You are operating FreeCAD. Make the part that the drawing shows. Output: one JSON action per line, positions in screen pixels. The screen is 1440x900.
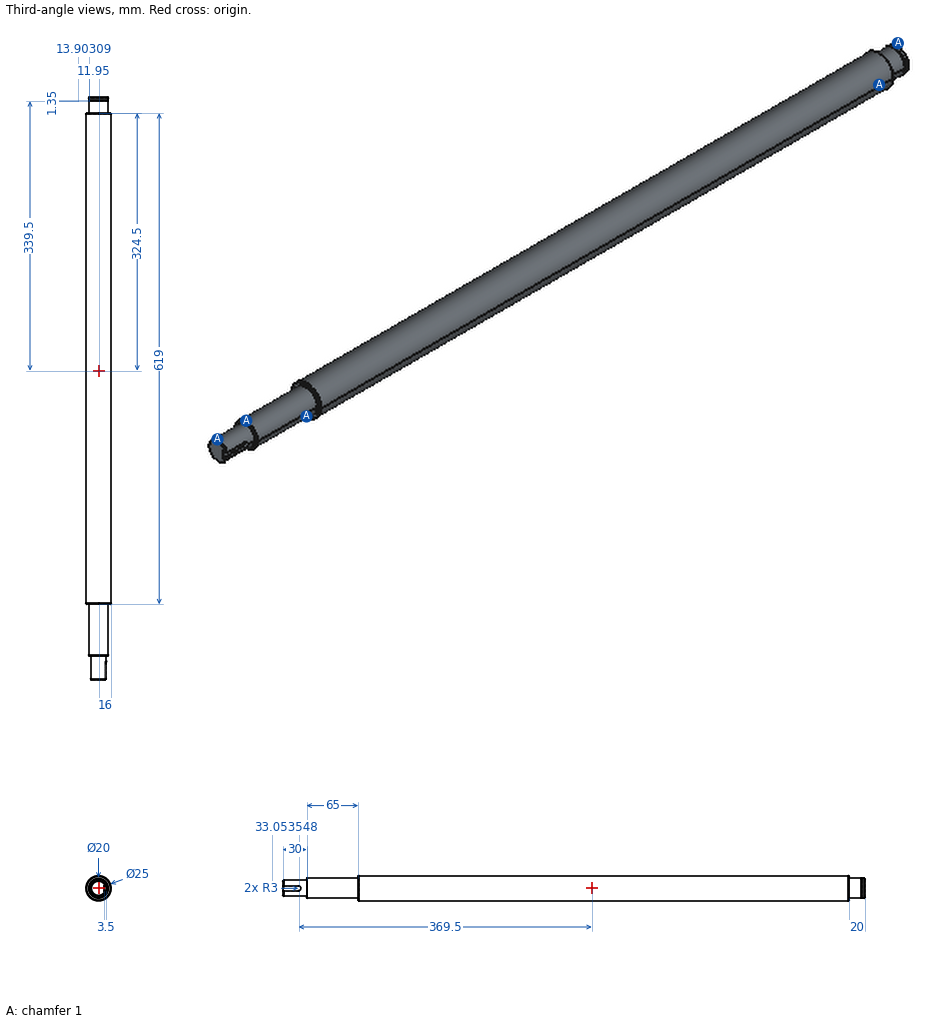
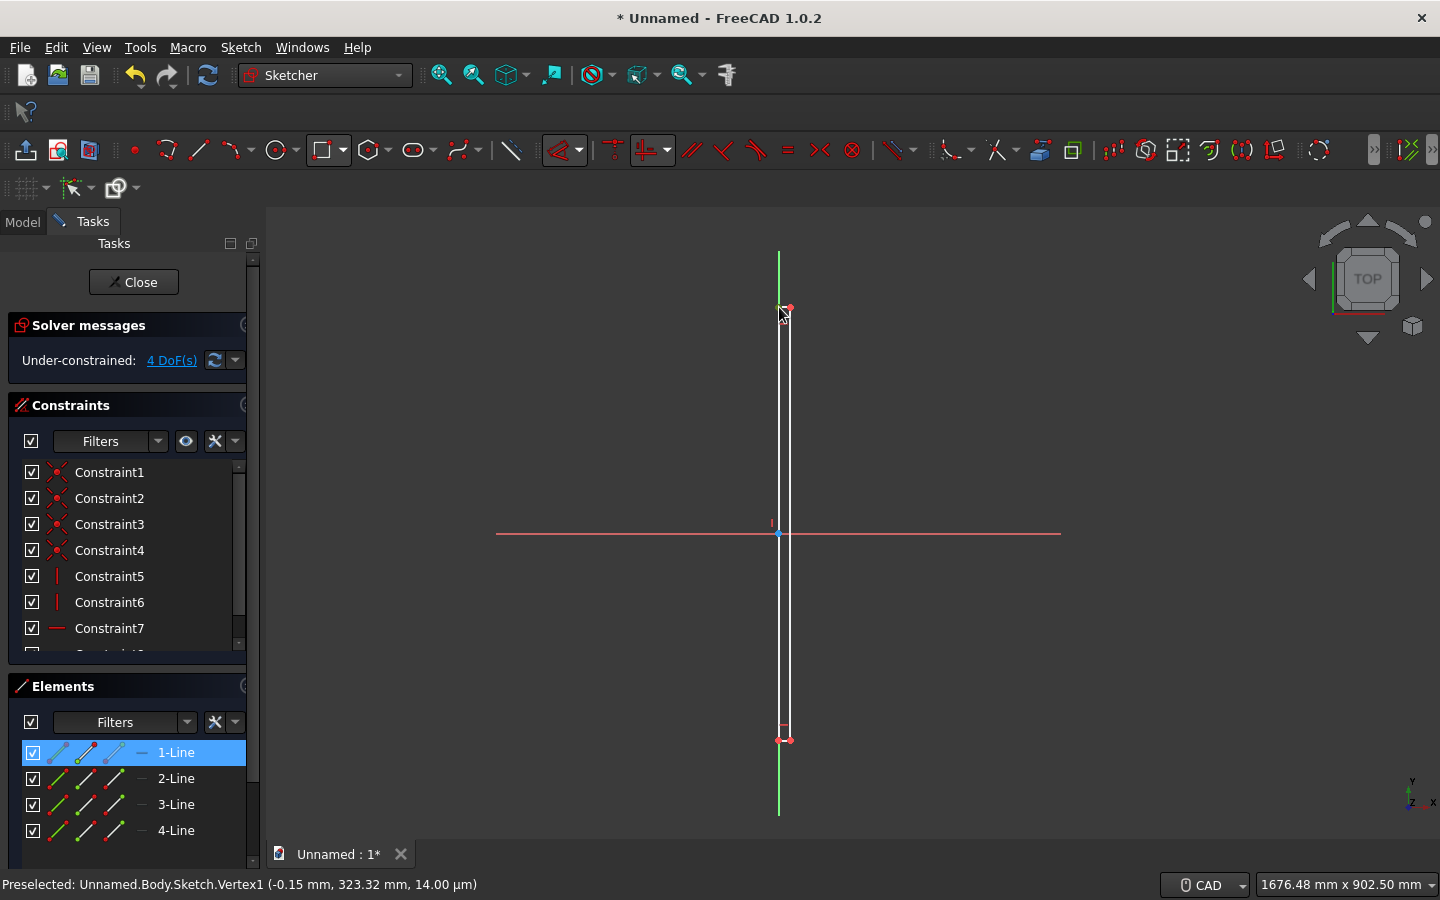
{"action": "left_click", "coordinate": [779, 276]}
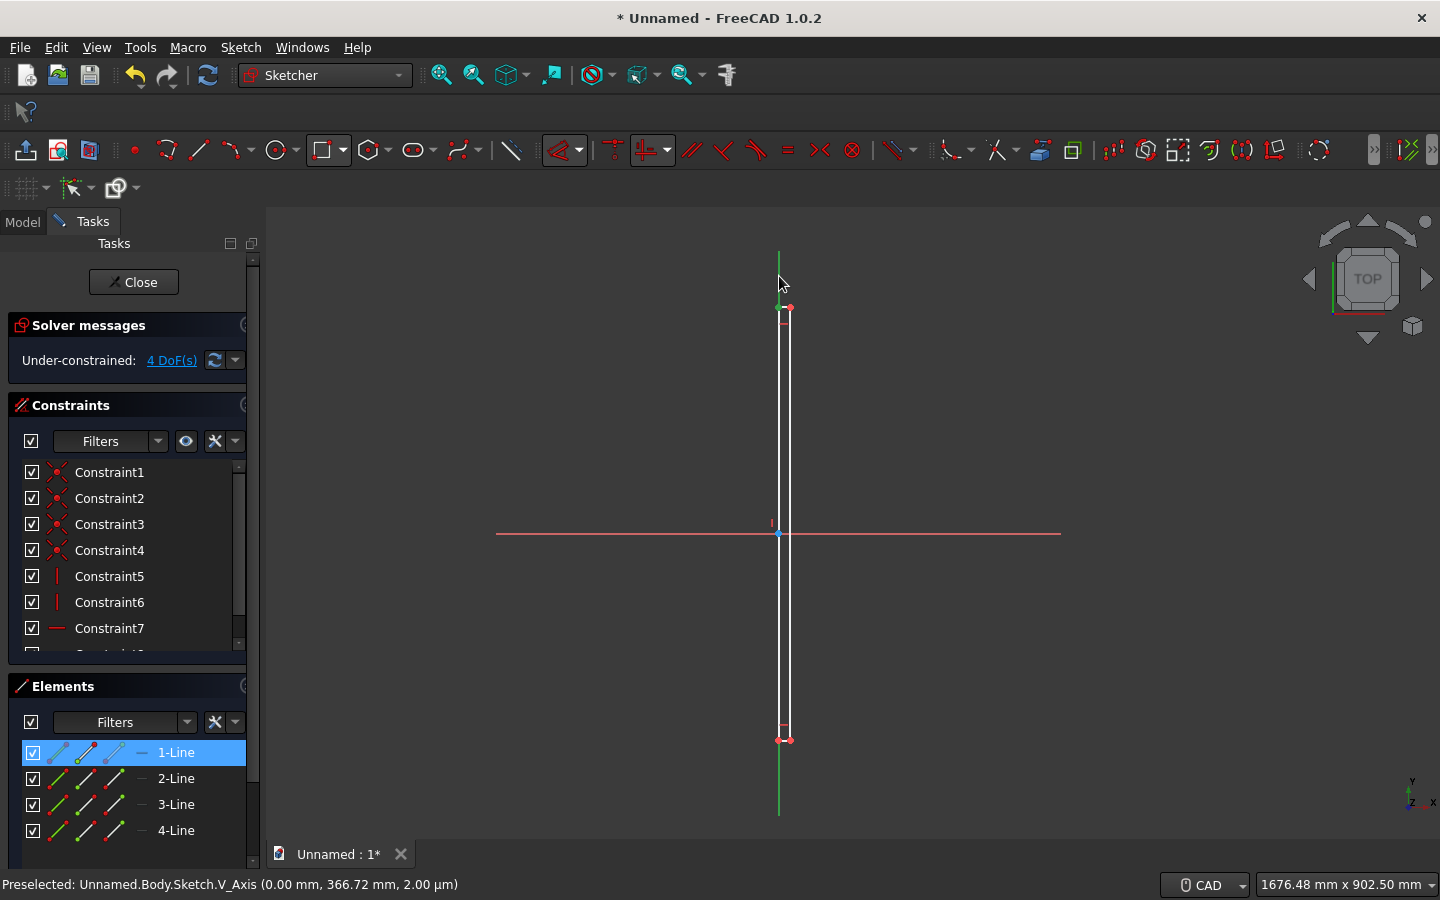
{"action": "left_click", "coordinate": [614, 150]}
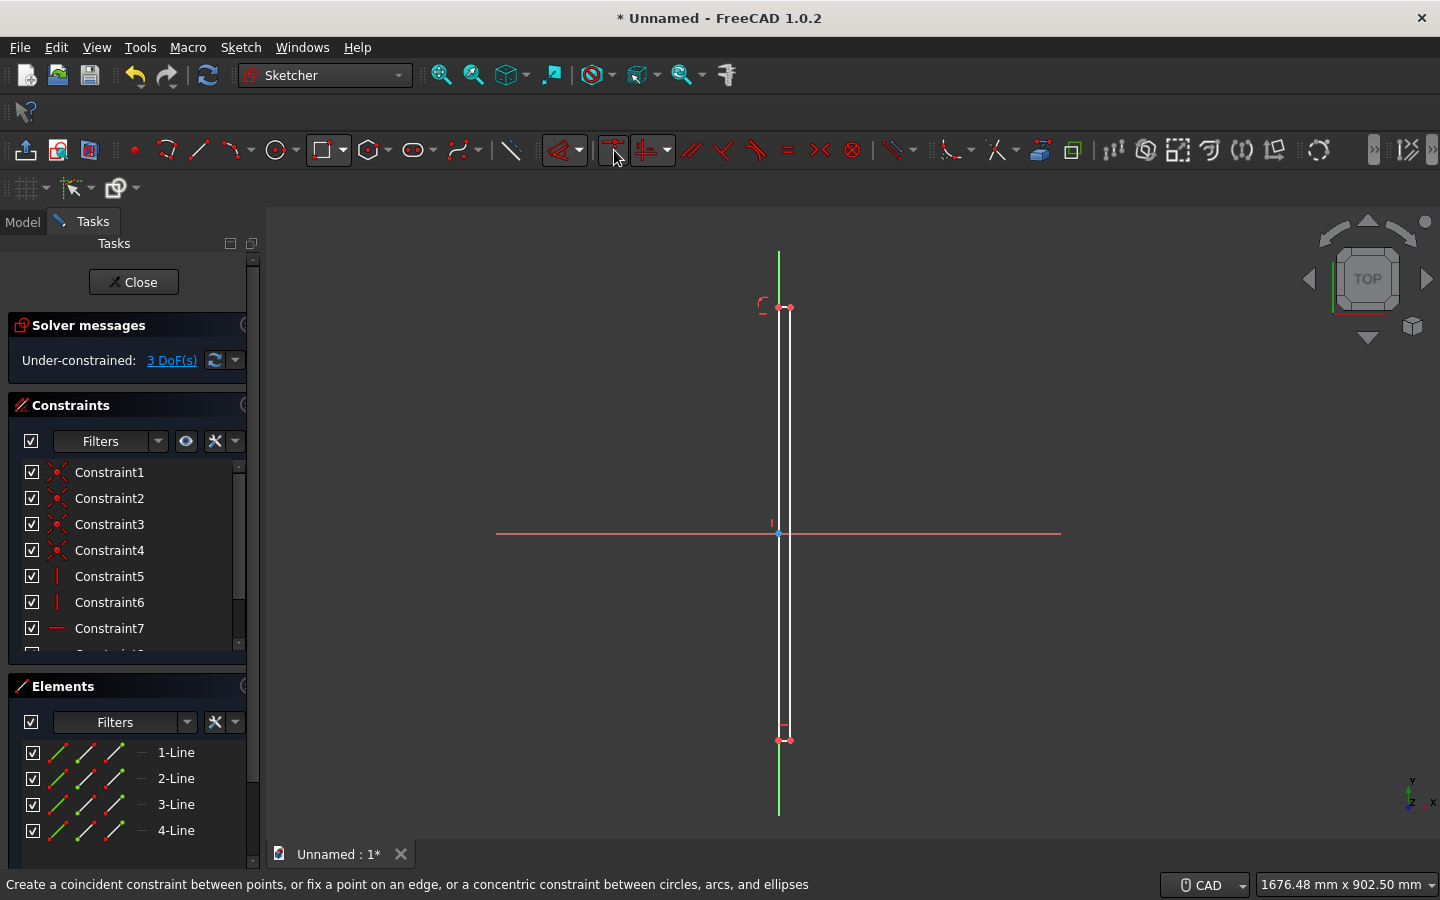
{"action": "left_click", "coordinate": [558, 150]}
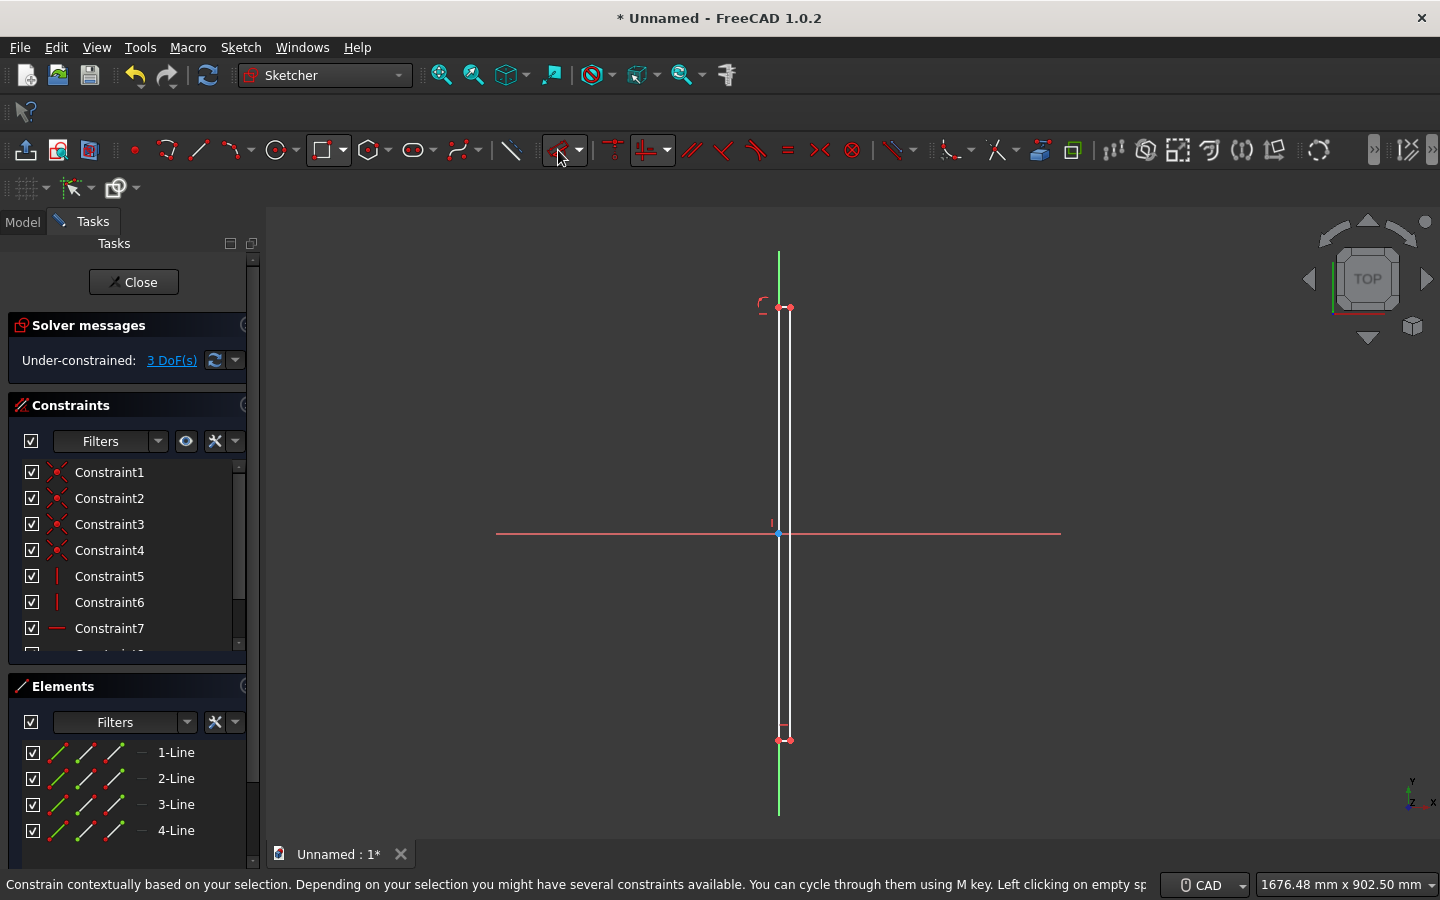
{"action": "scroll", "coordinate": [785, 741], "scroll_direction": "up", "scroll_amount": 7}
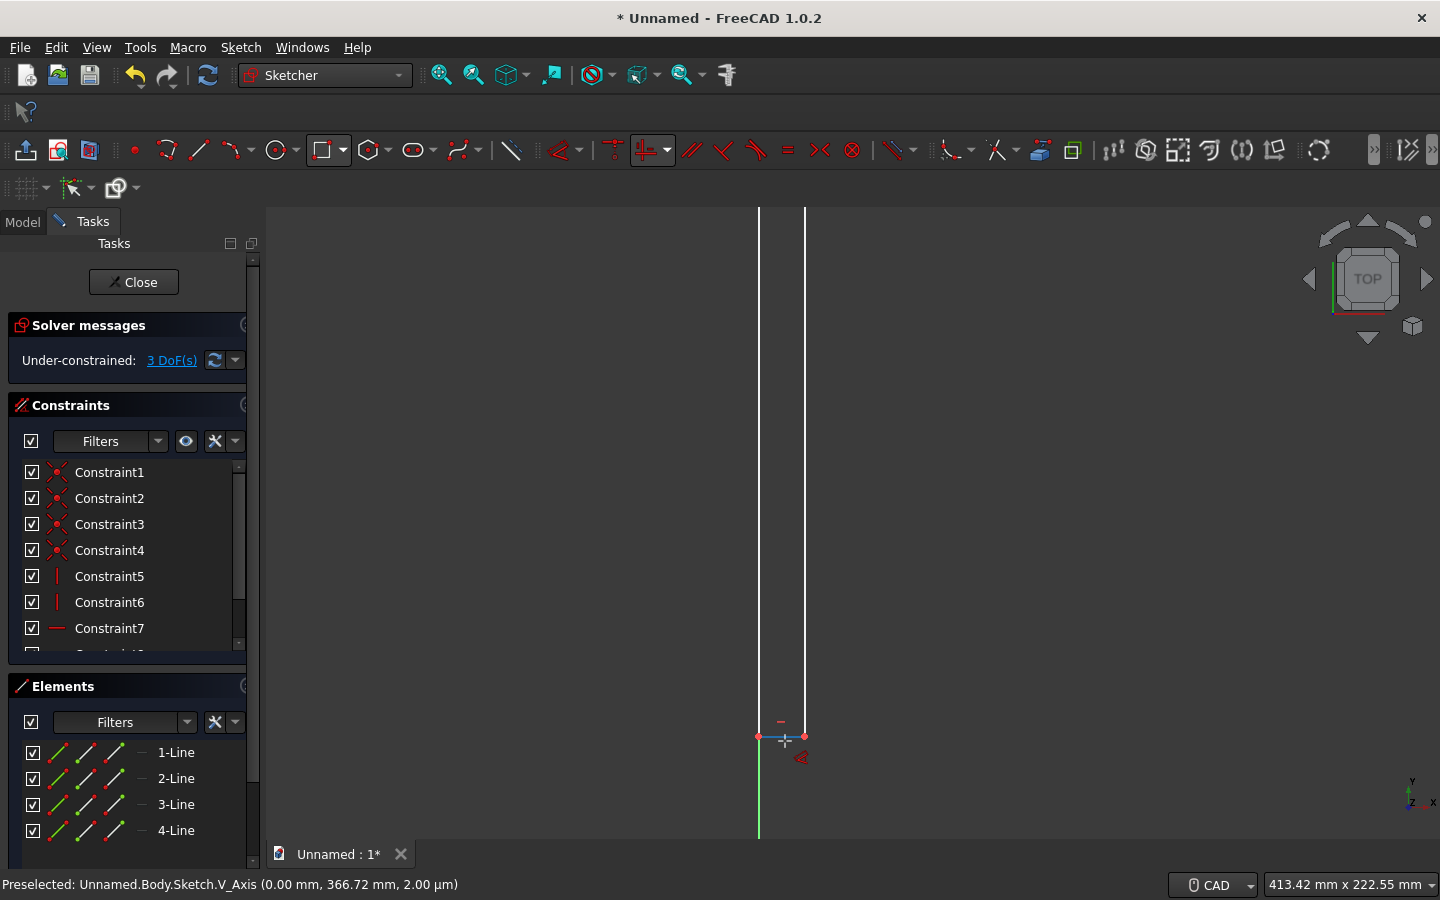
{"action": "left_click", "coordinate": [782, 737]}
{"action": "left_click", "coordinate": [782, 771]}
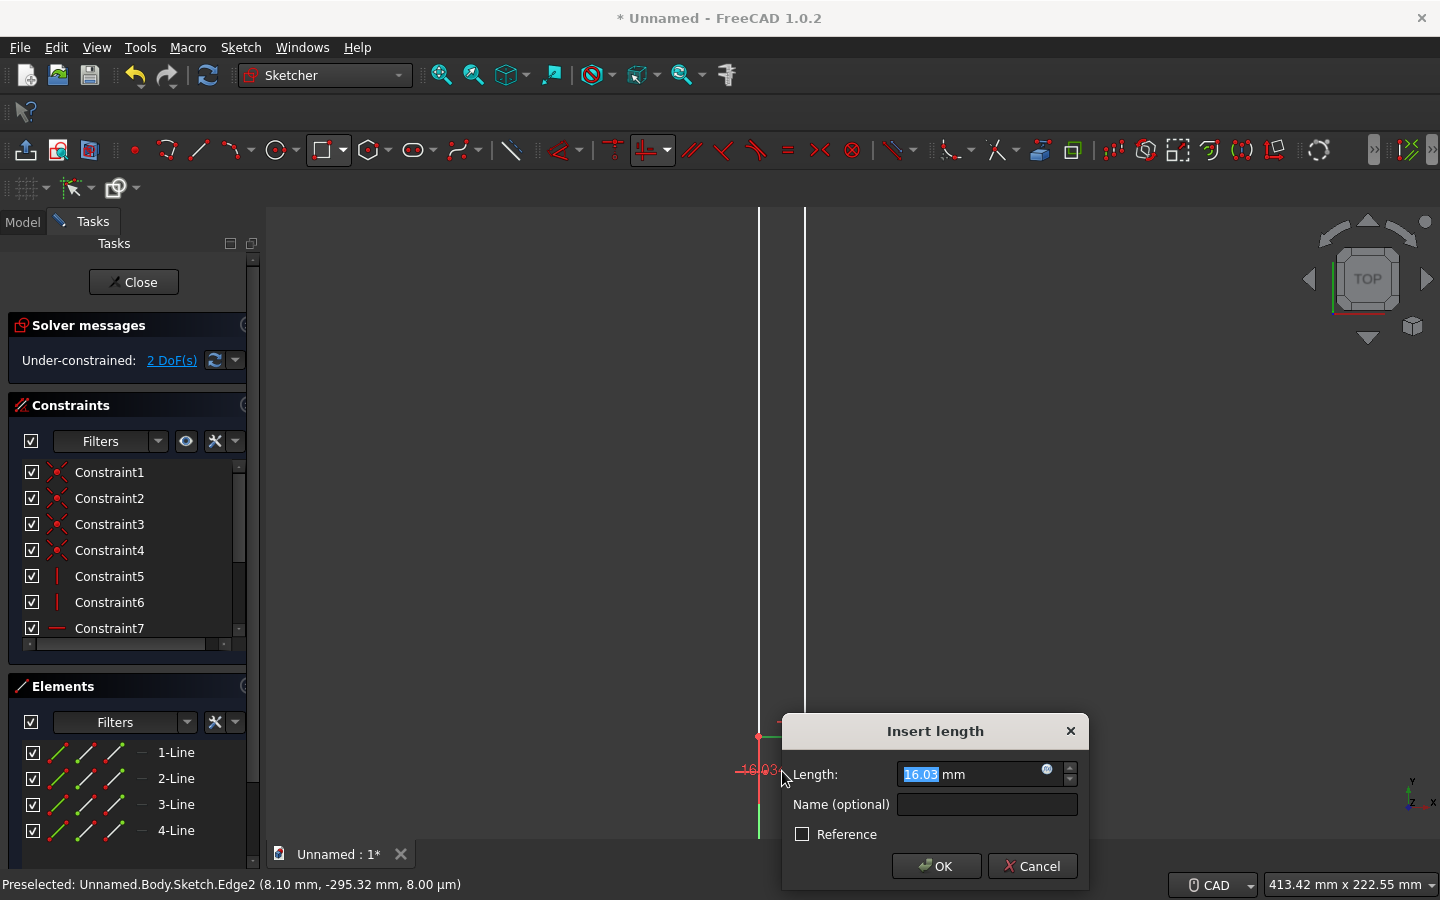
{"action": "type", "text": "16"}
{"action": "key", "text": "Return"}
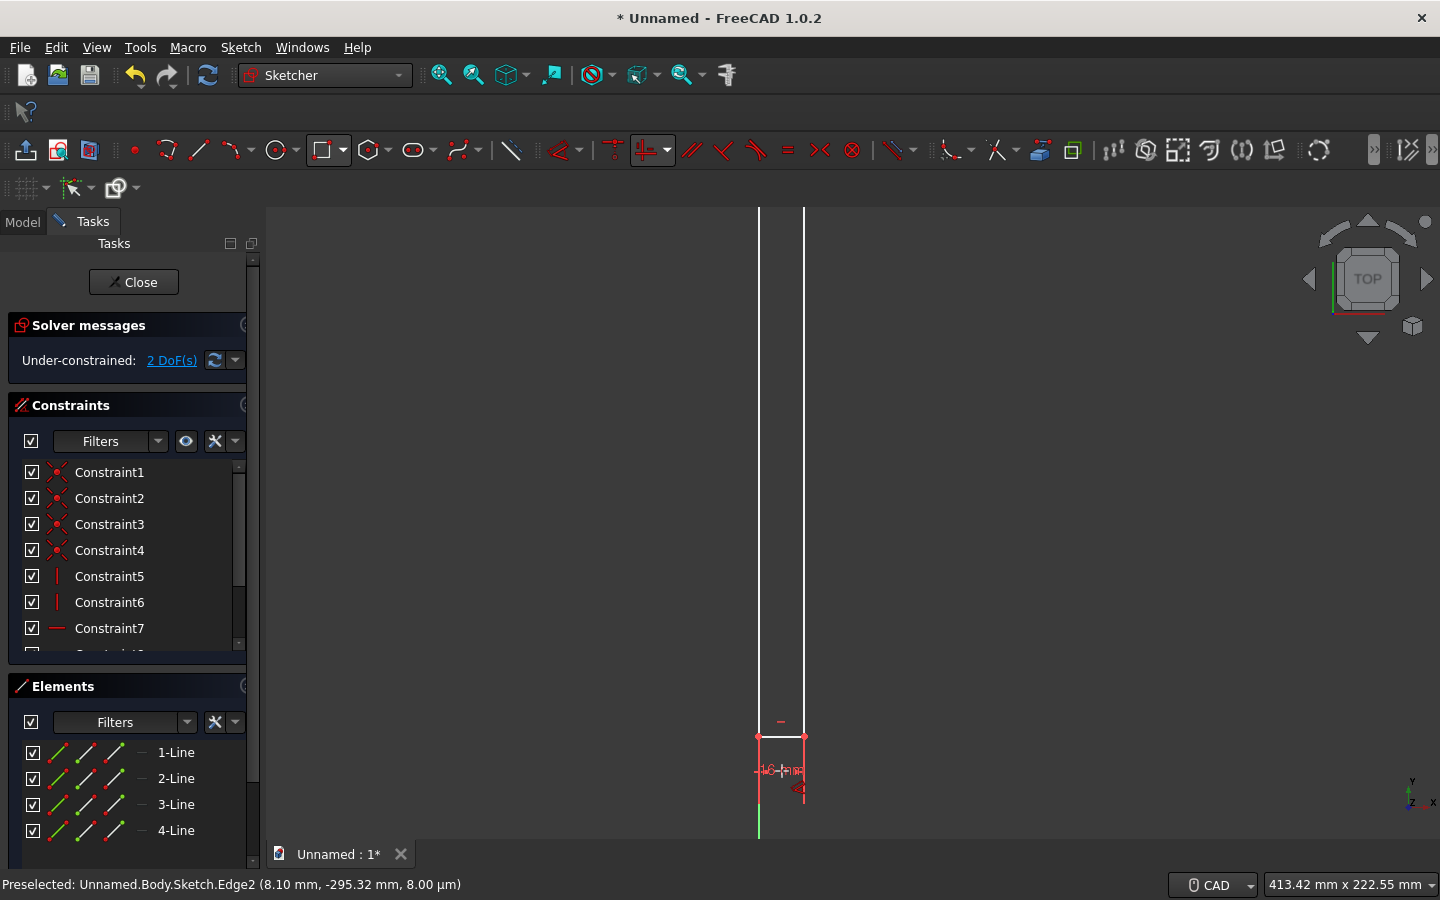
{"action": "scroll", "coordinate": [785, 741], "scroll_direction": "down", "scroll_amount": 7}